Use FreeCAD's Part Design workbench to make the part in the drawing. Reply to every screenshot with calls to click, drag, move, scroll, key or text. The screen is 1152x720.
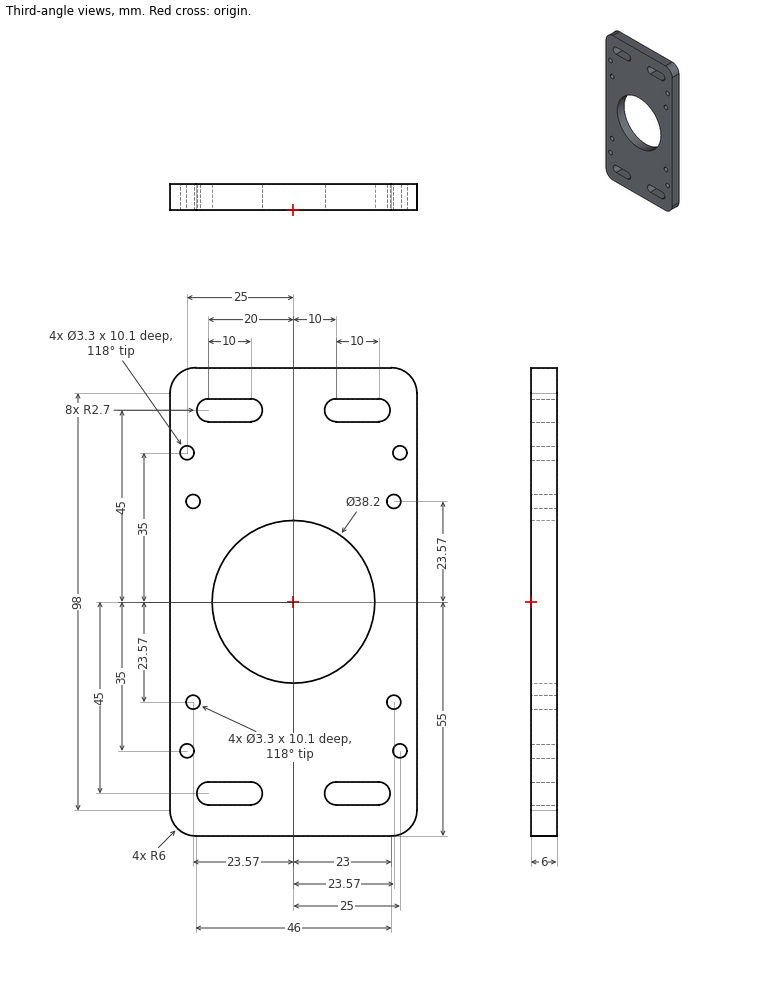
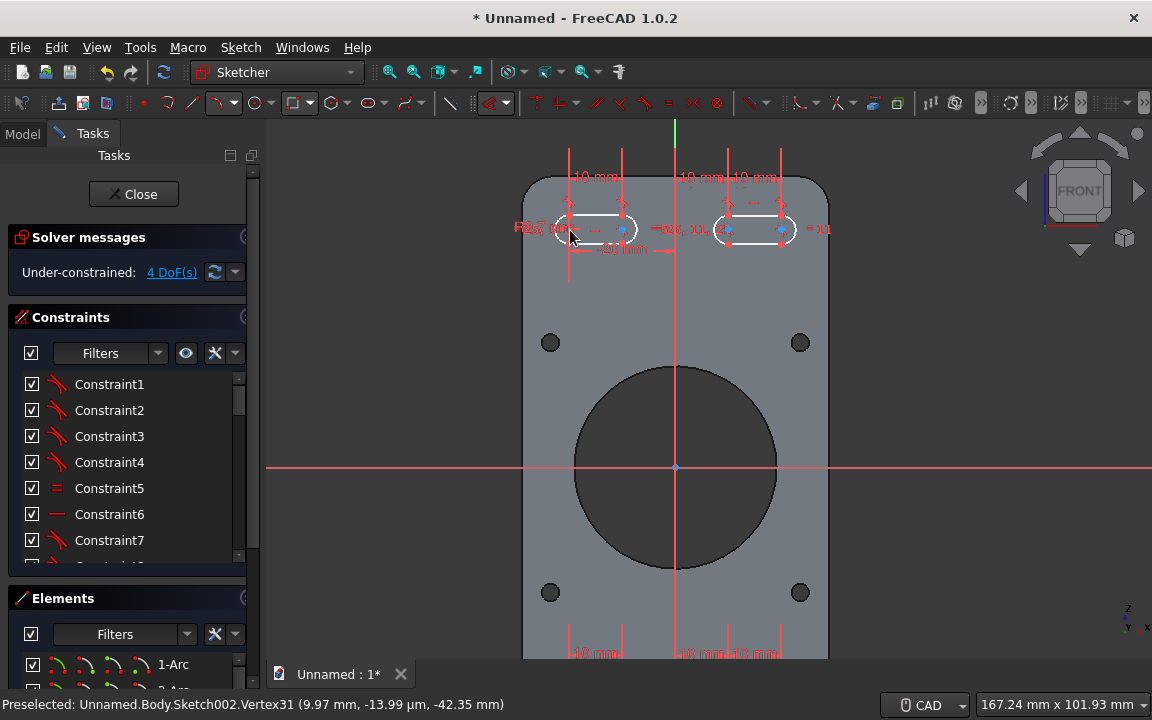
click(569, 229)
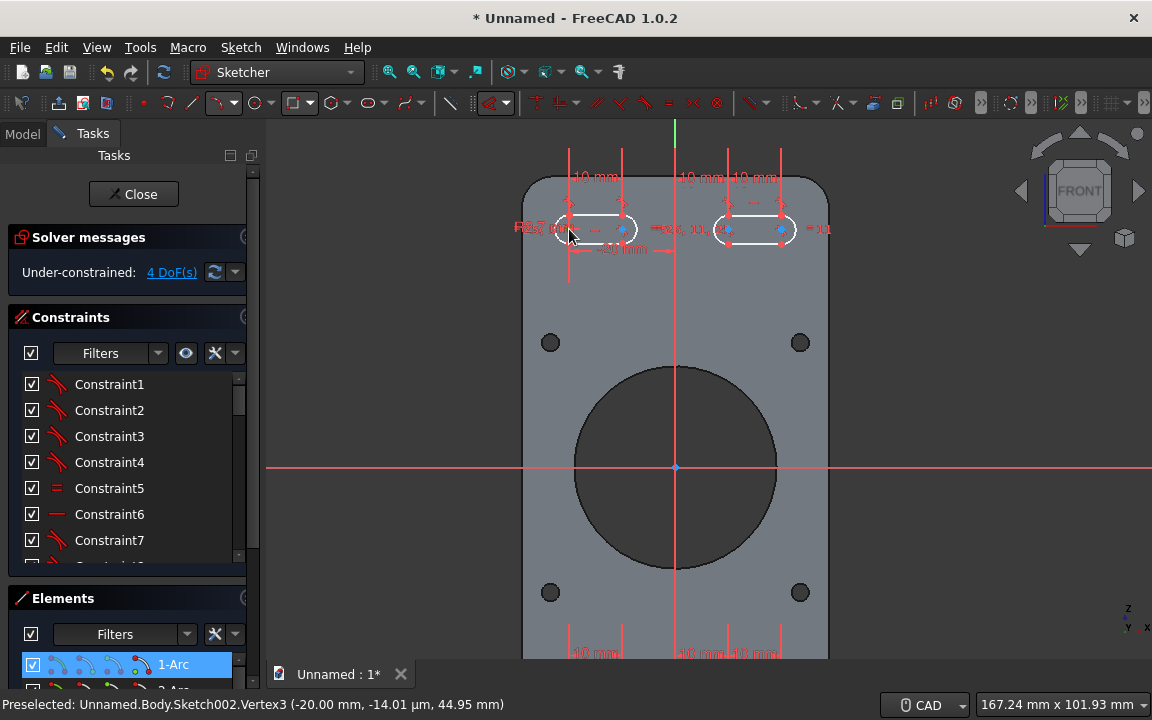
key(i)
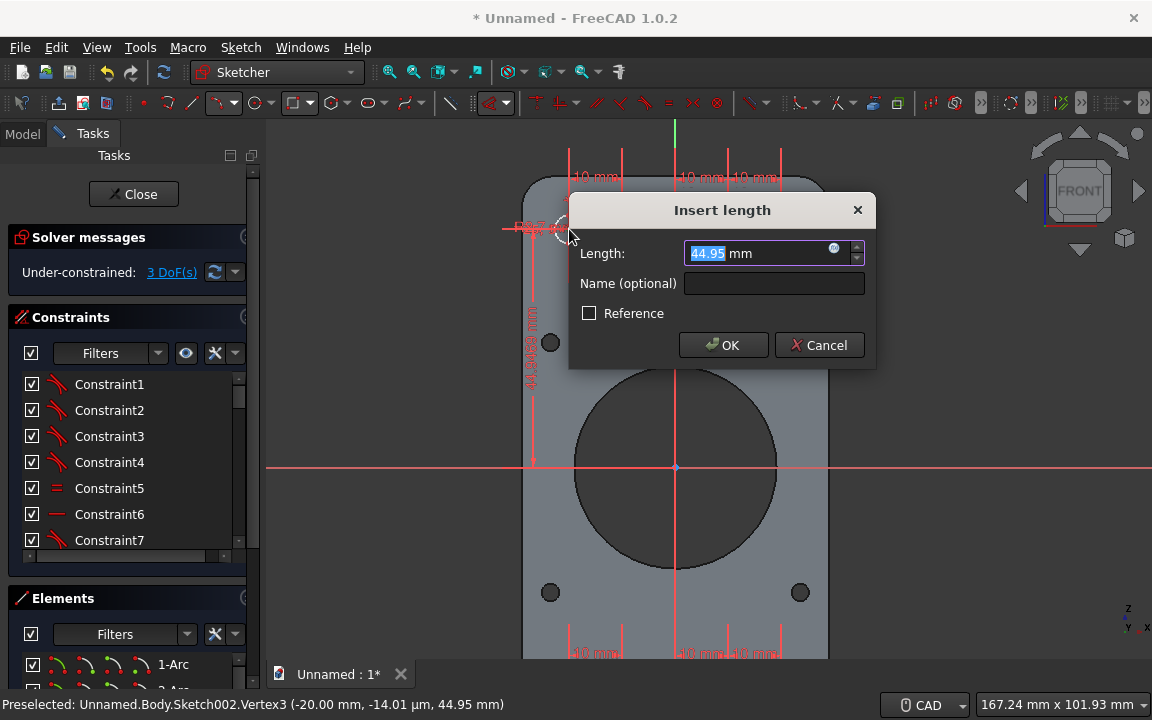
text(45)
key(Return)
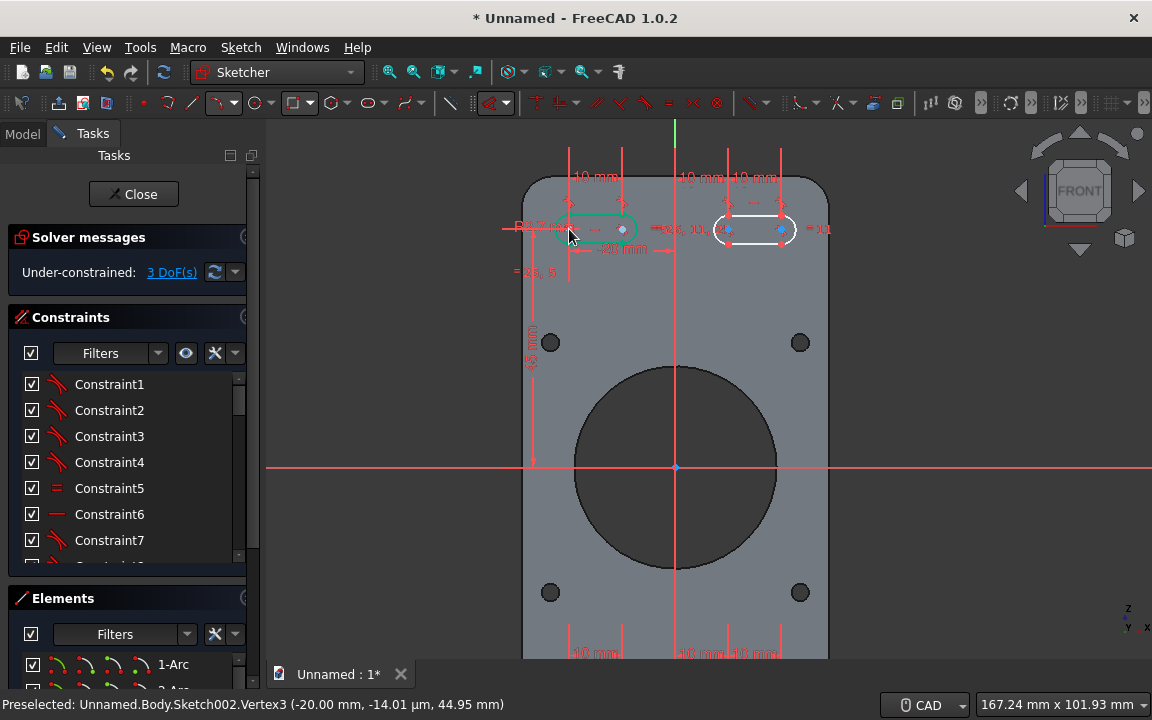
click(728, 230)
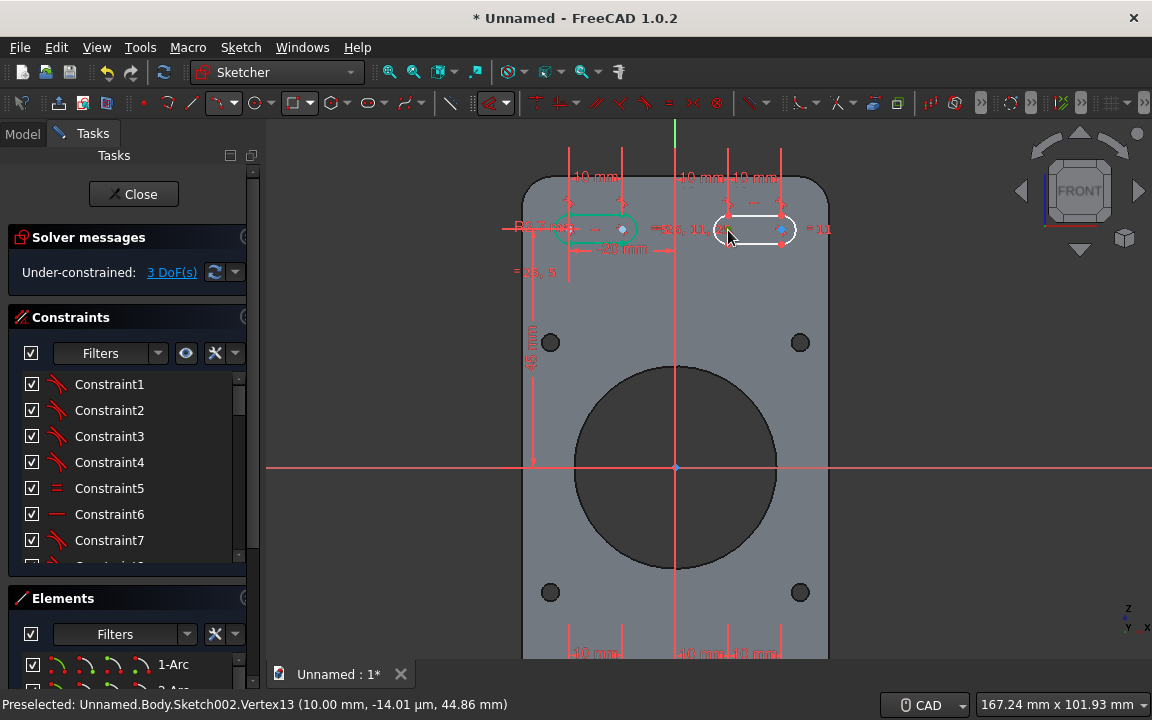
key(i)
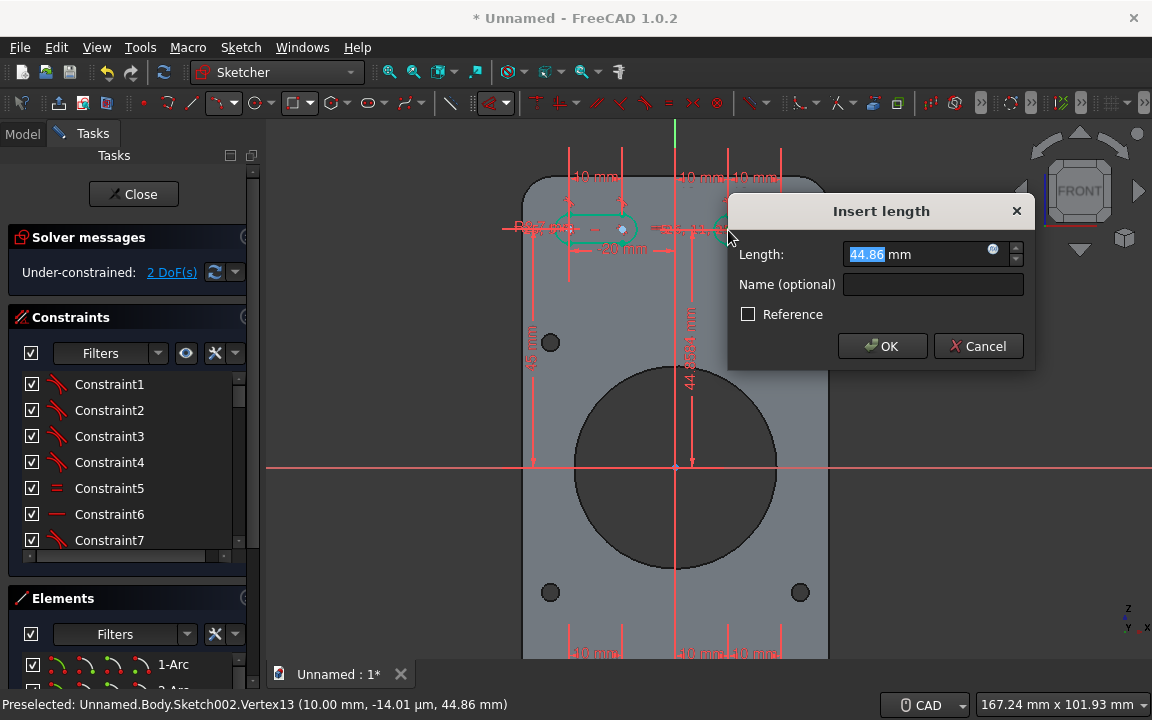
text(45)
key(Return)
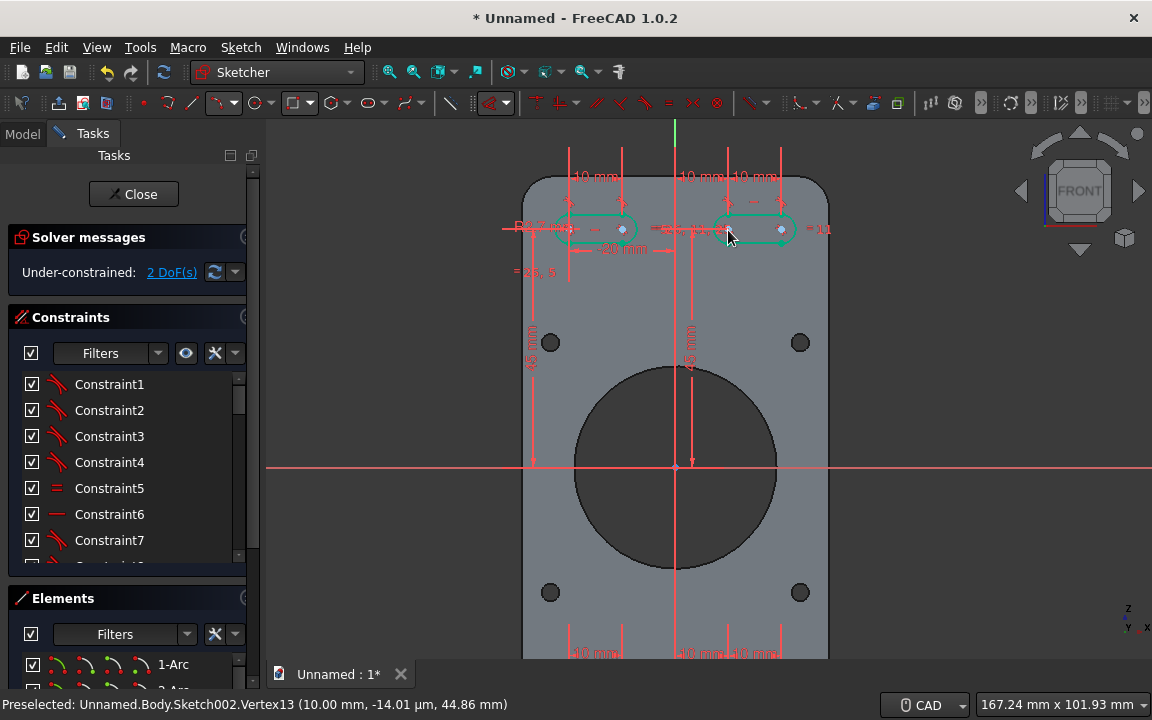
scroll(570, 229, down, 2)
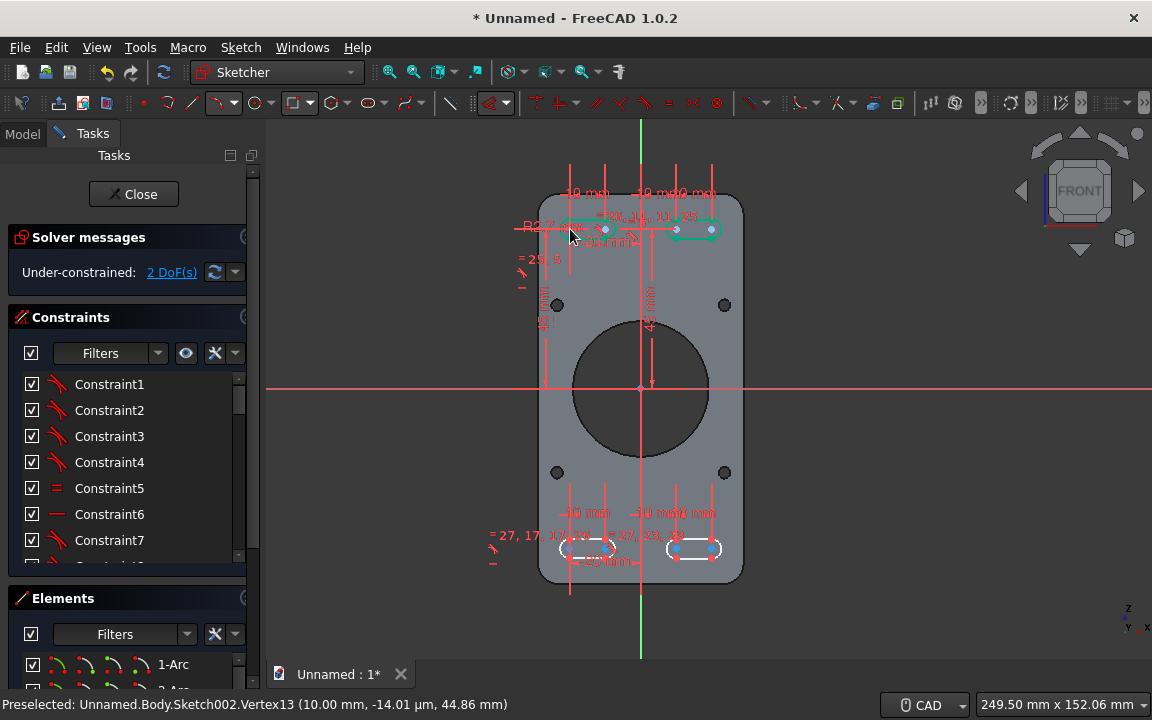
scroll(570, 549, up, 2)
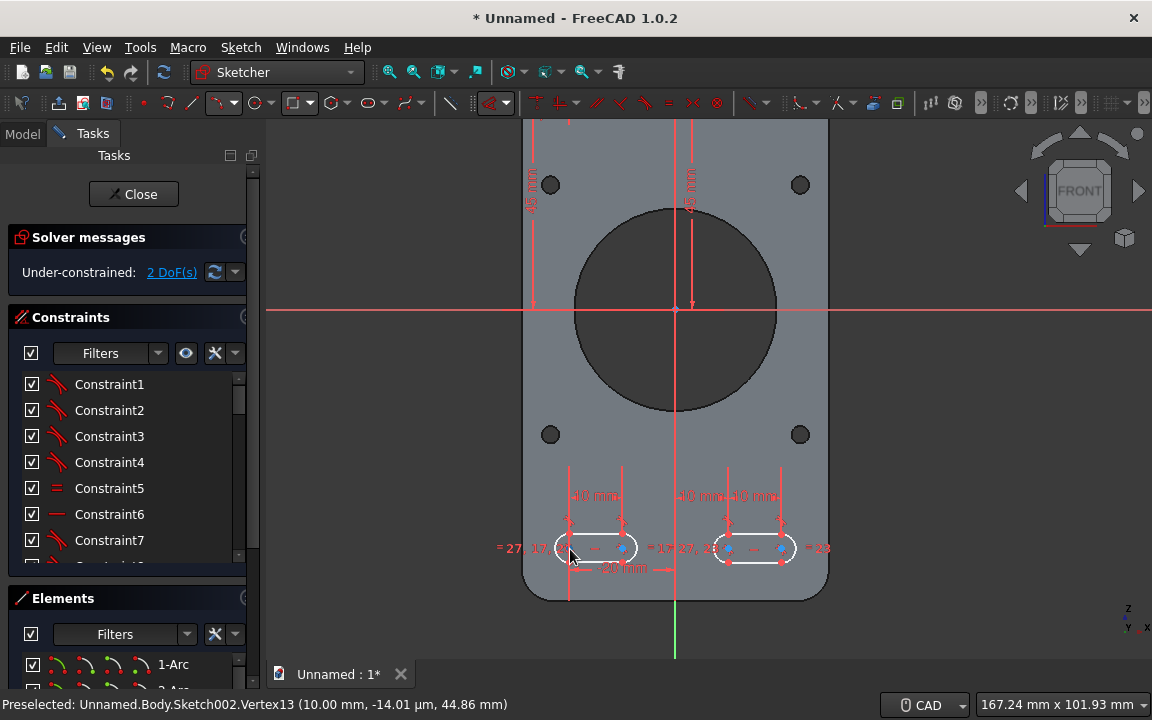
click(569, 548)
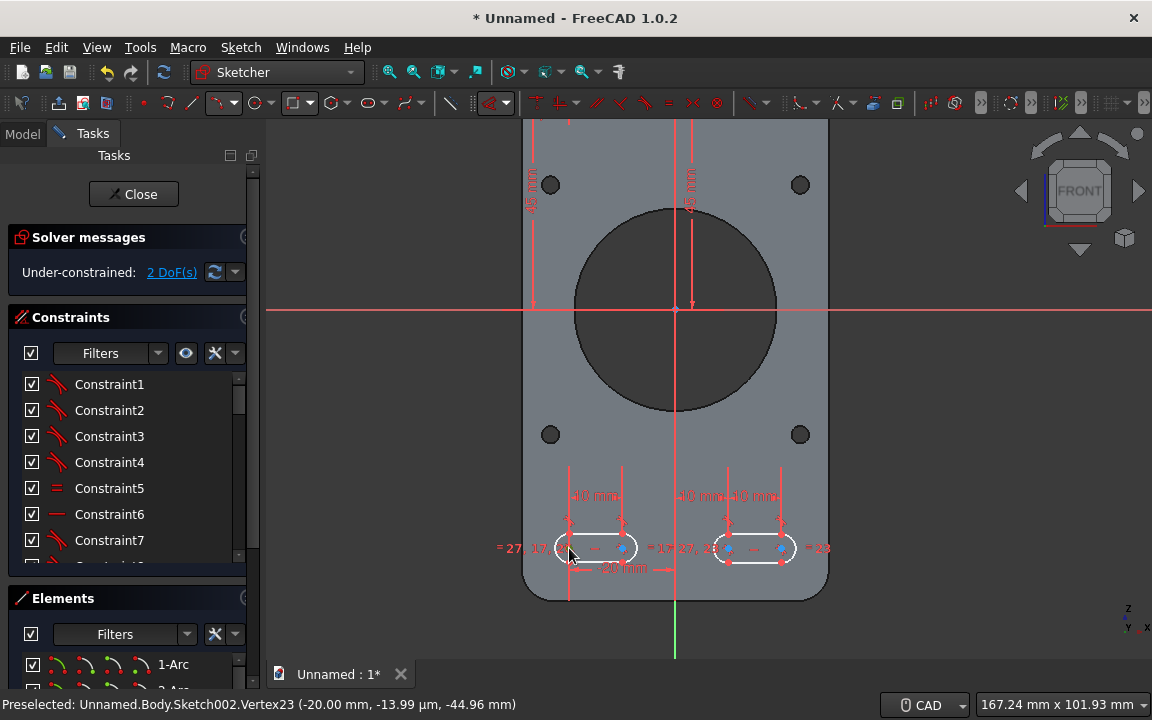
click(508, 104)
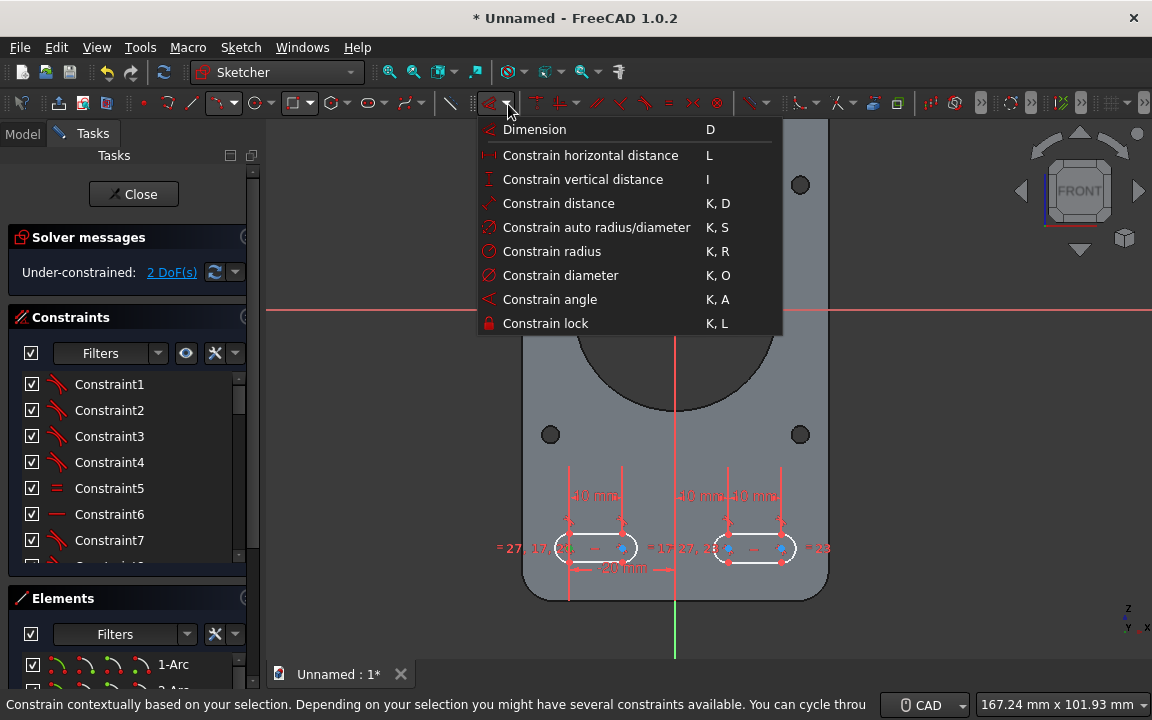
click(630, 179)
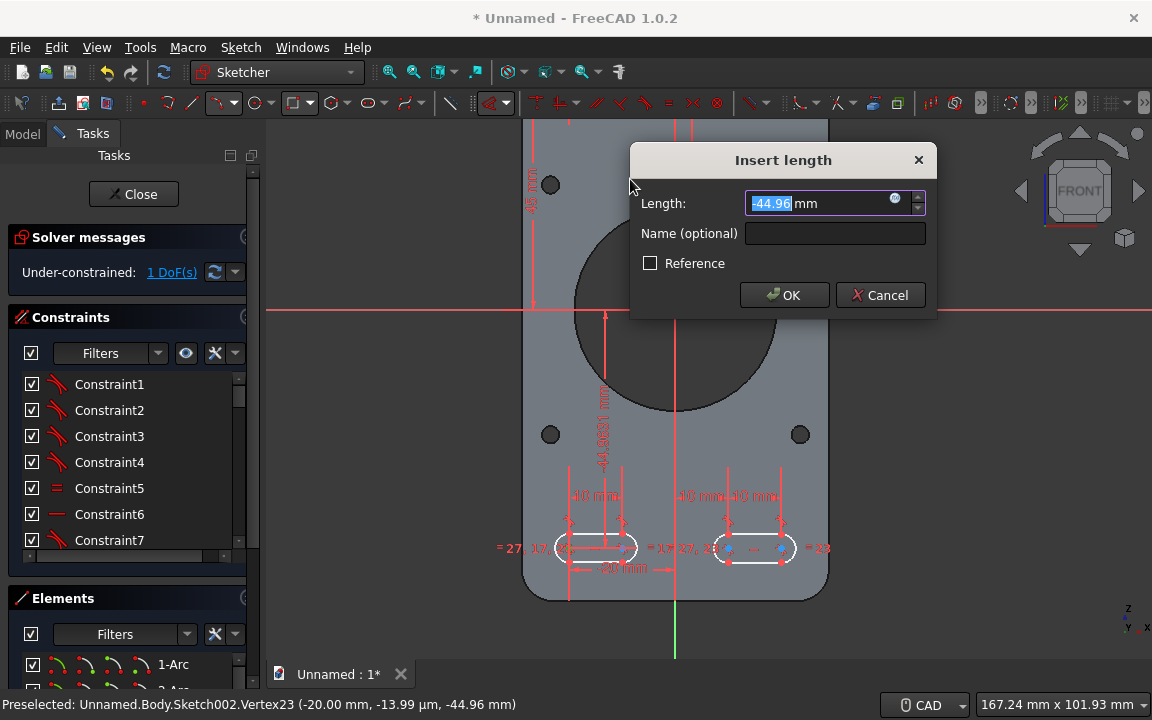
text(-45)
key(Return)